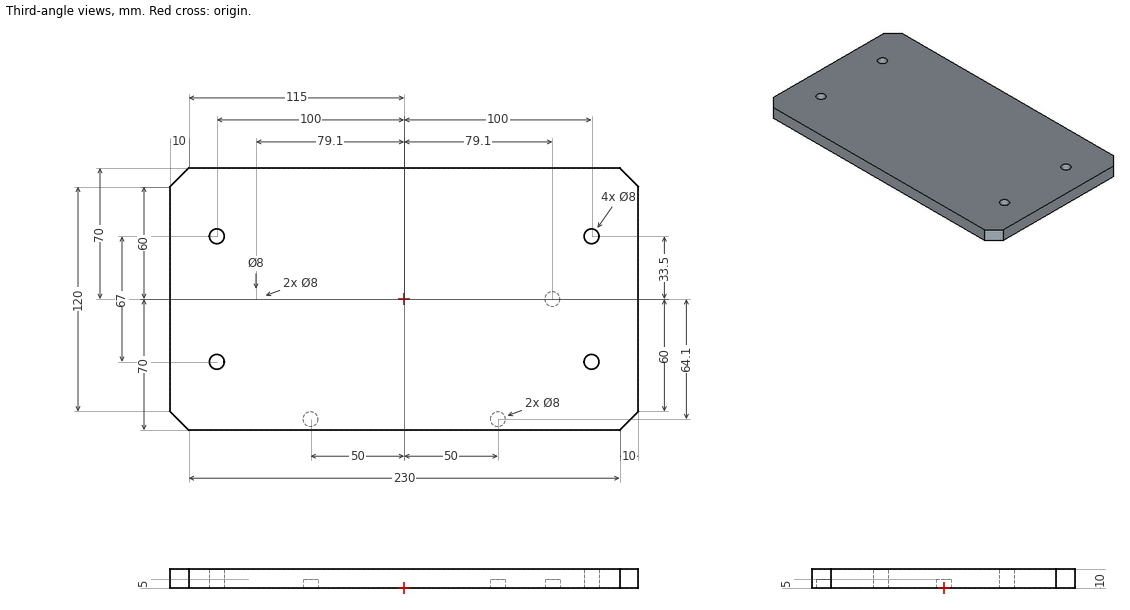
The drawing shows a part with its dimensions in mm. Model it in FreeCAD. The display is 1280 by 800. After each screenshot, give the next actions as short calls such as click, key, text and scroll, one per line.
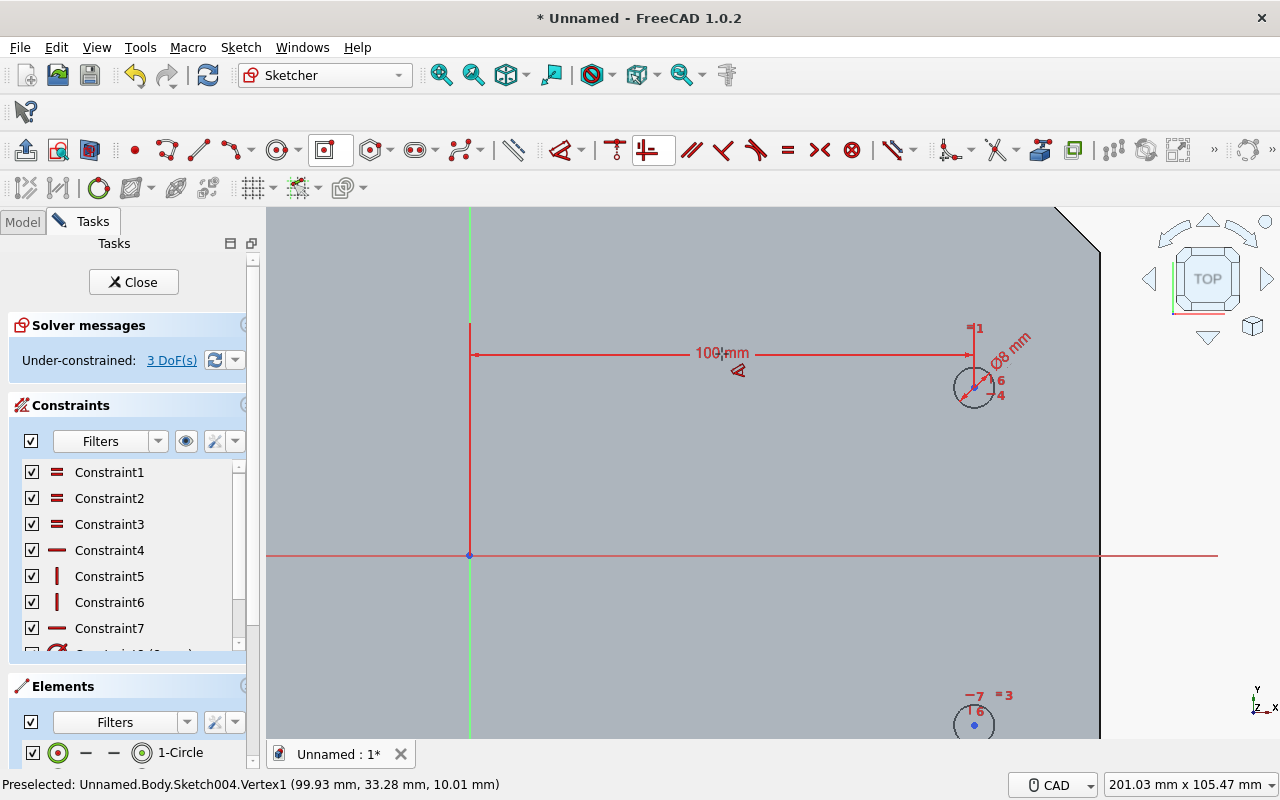
scroll(990, 373, down, 3)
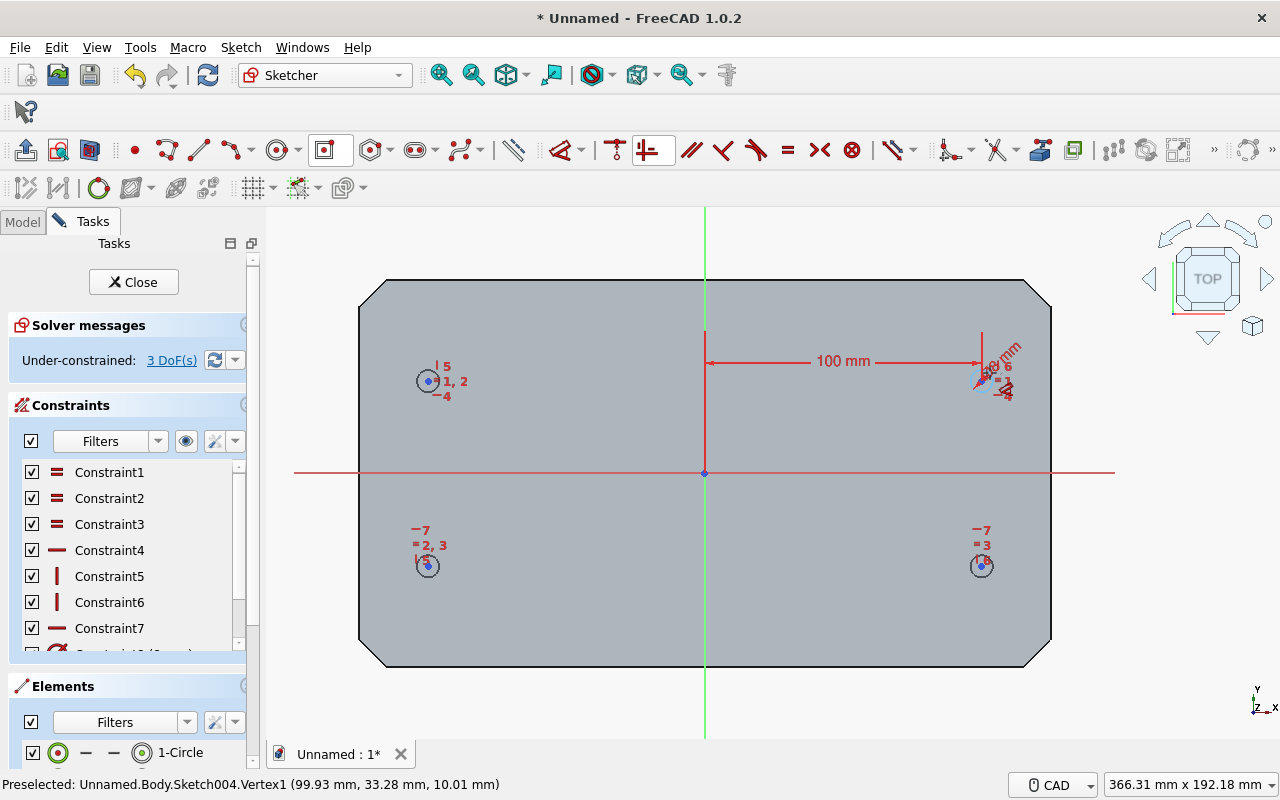
click(428, 381)
click(566, 347)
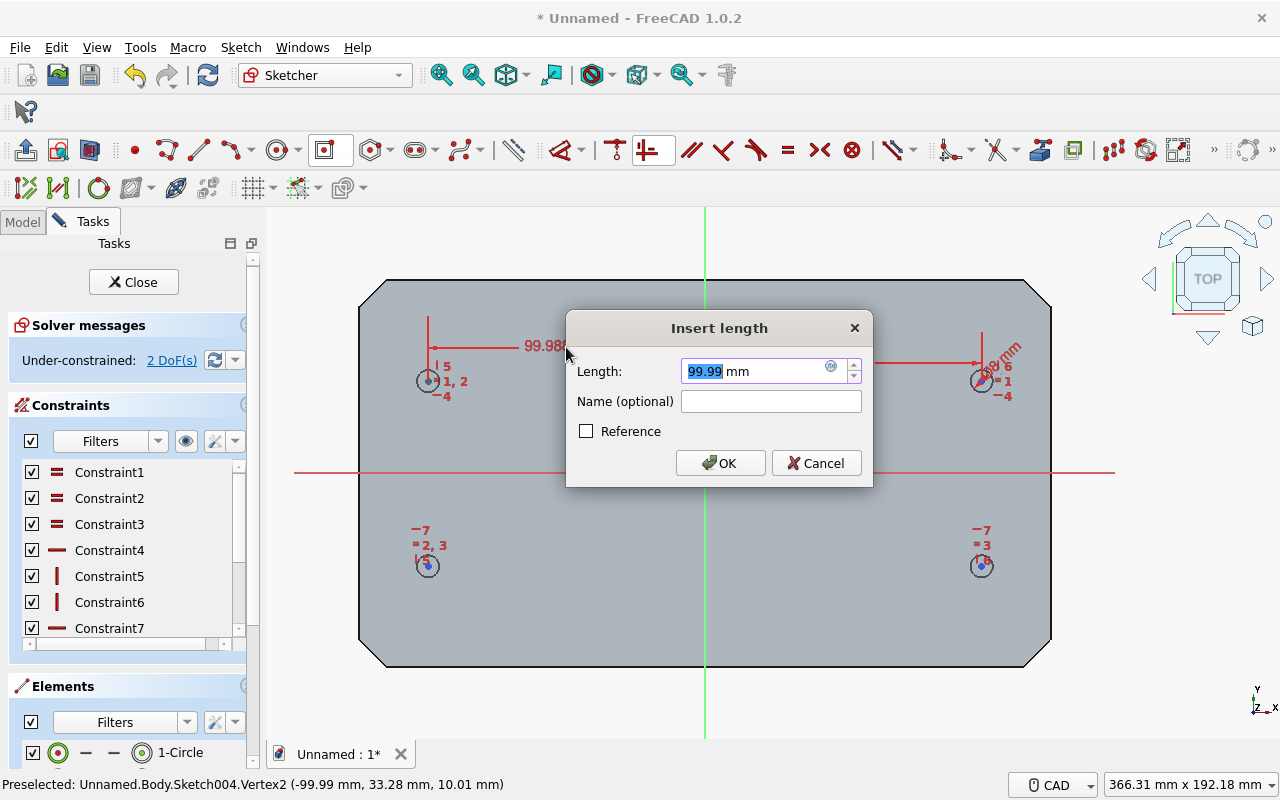
text(100)
key(Return)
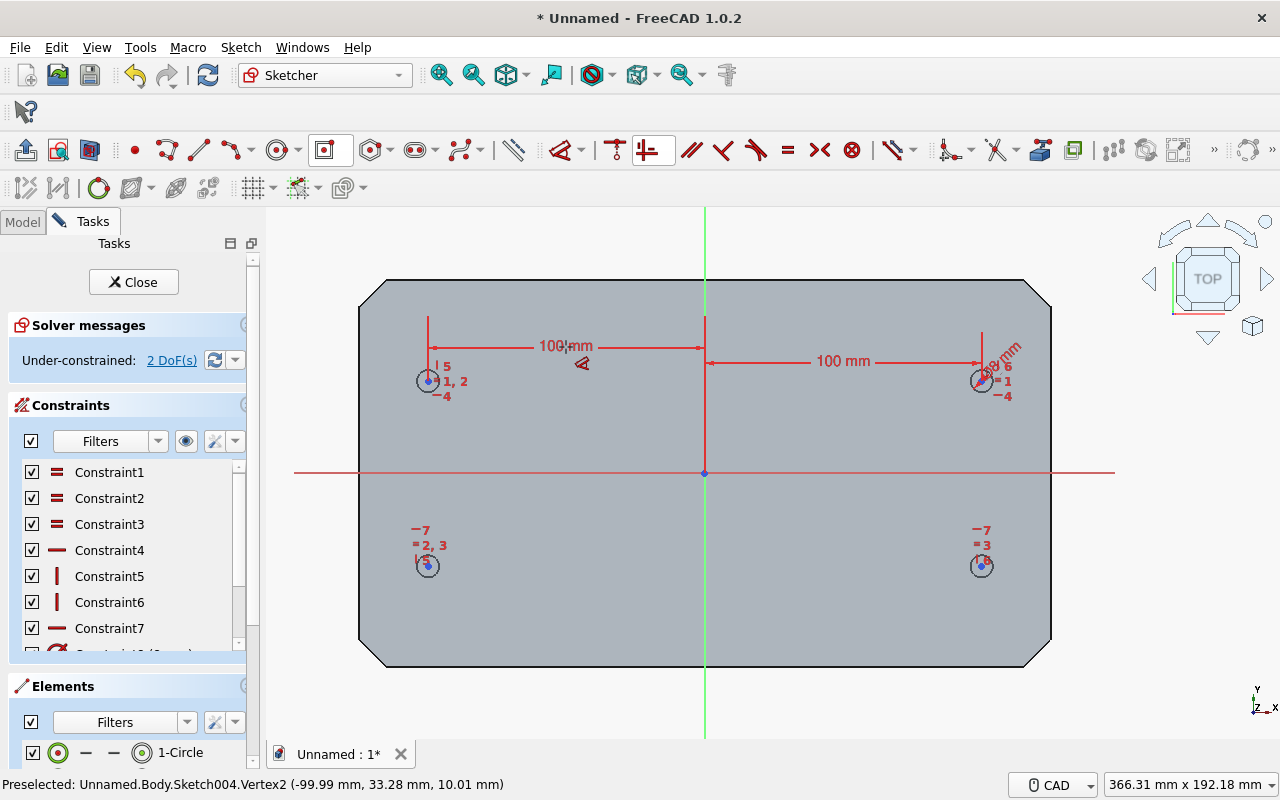
click(428, 381)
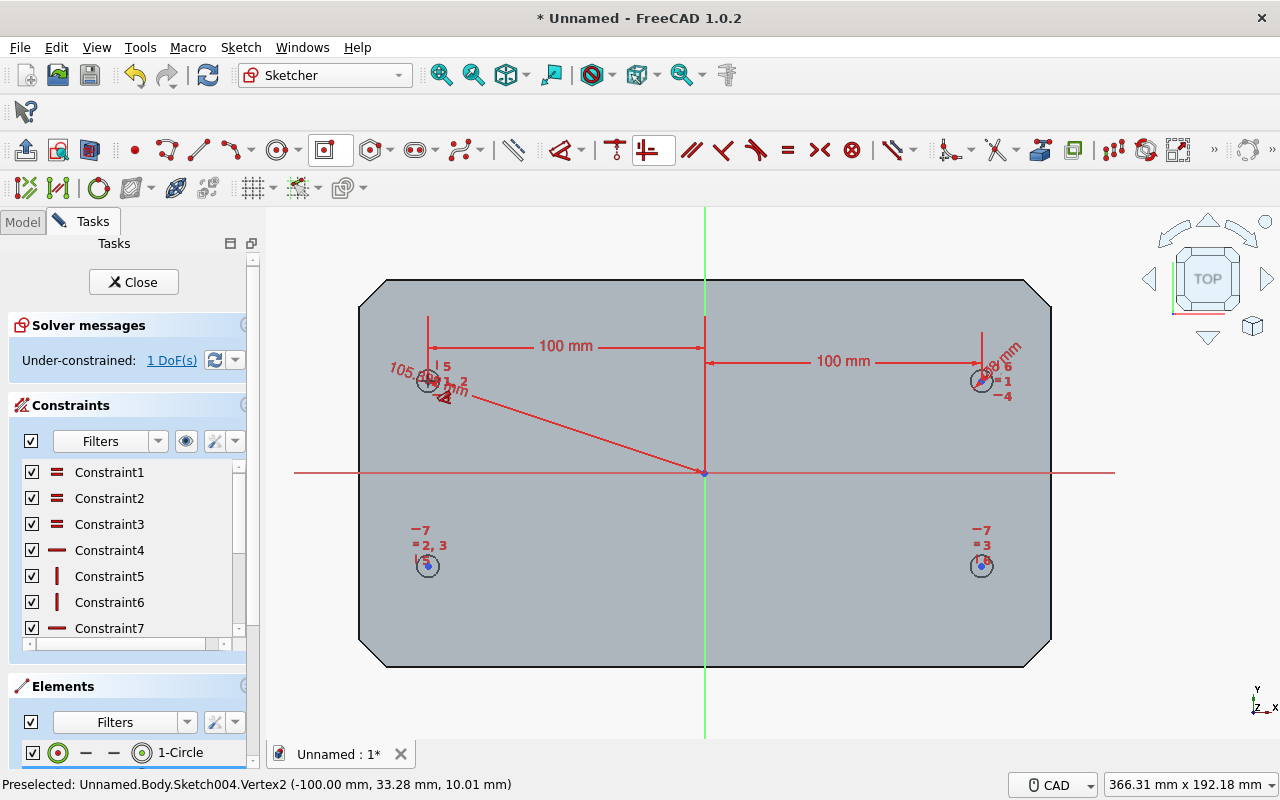
click(428, 566)
click(394, 431)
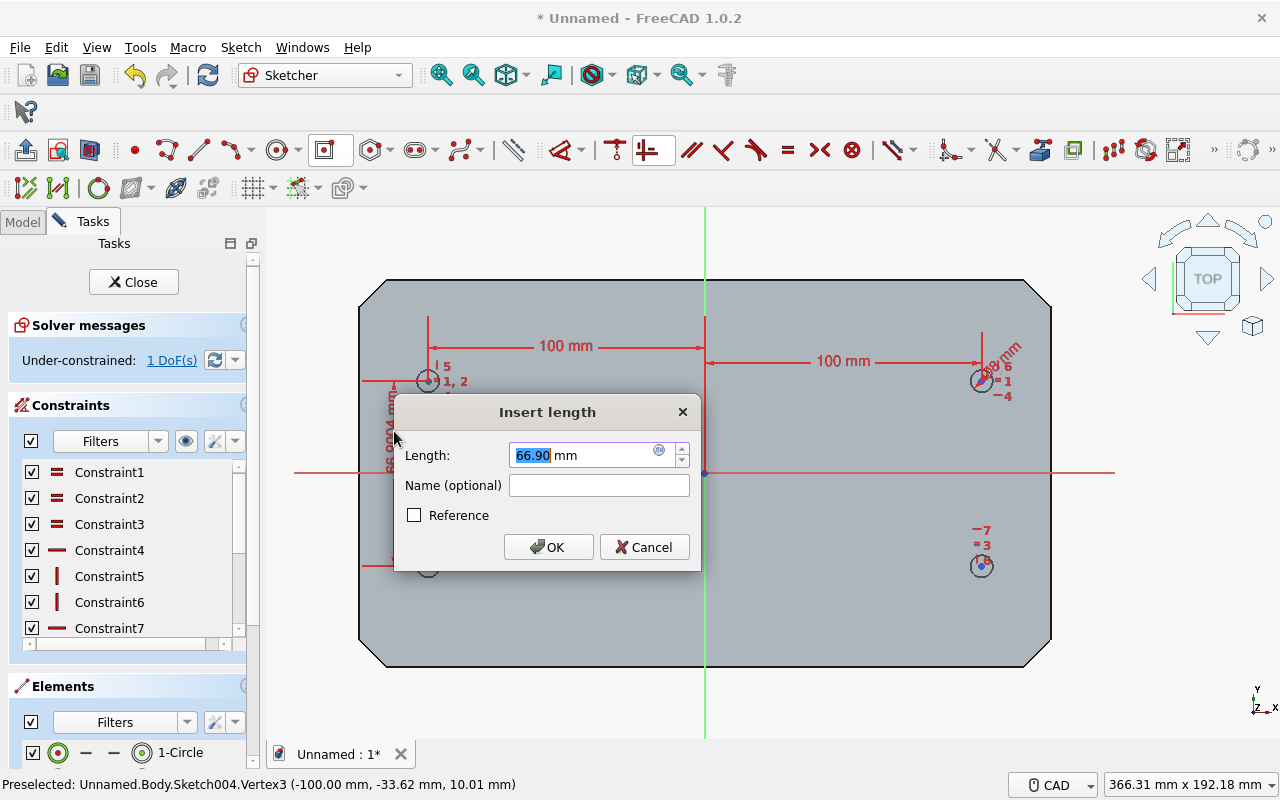
text(67)
key(Return)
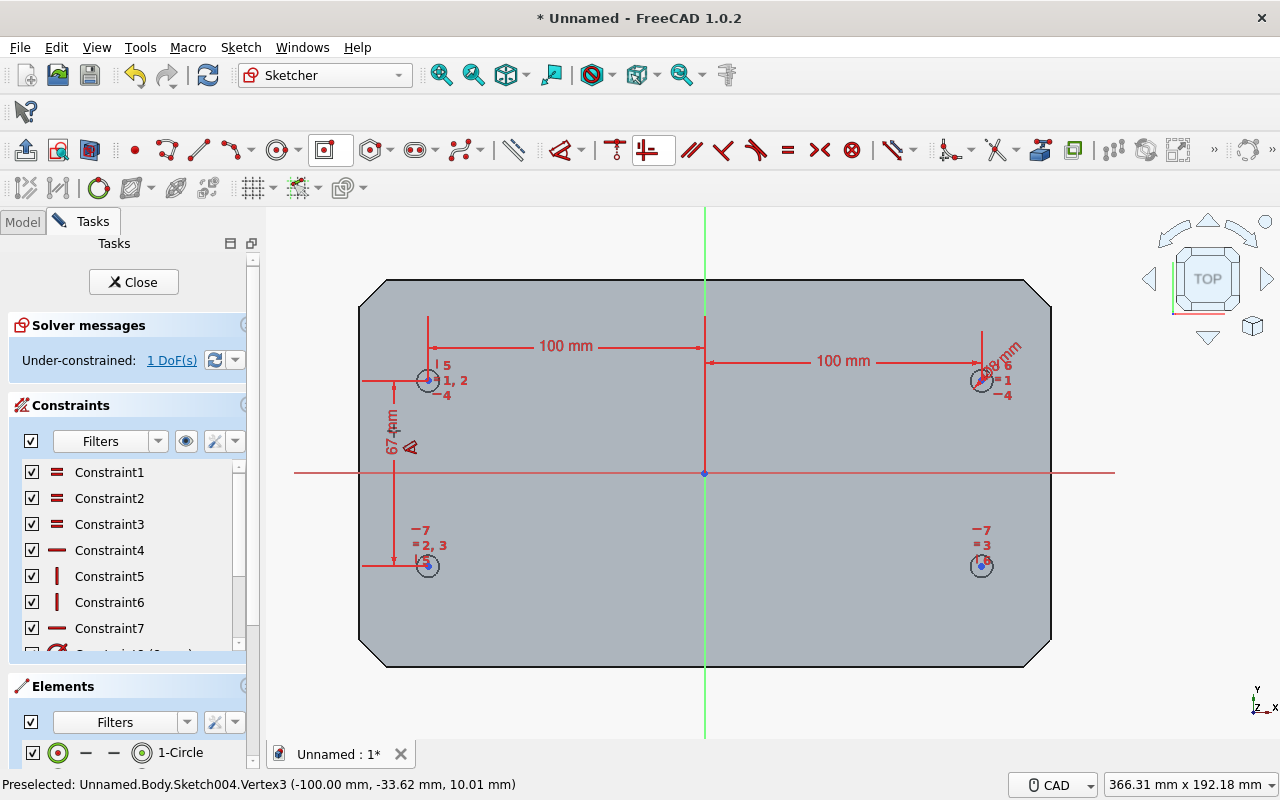
click(982, 381)
click(1016, 427)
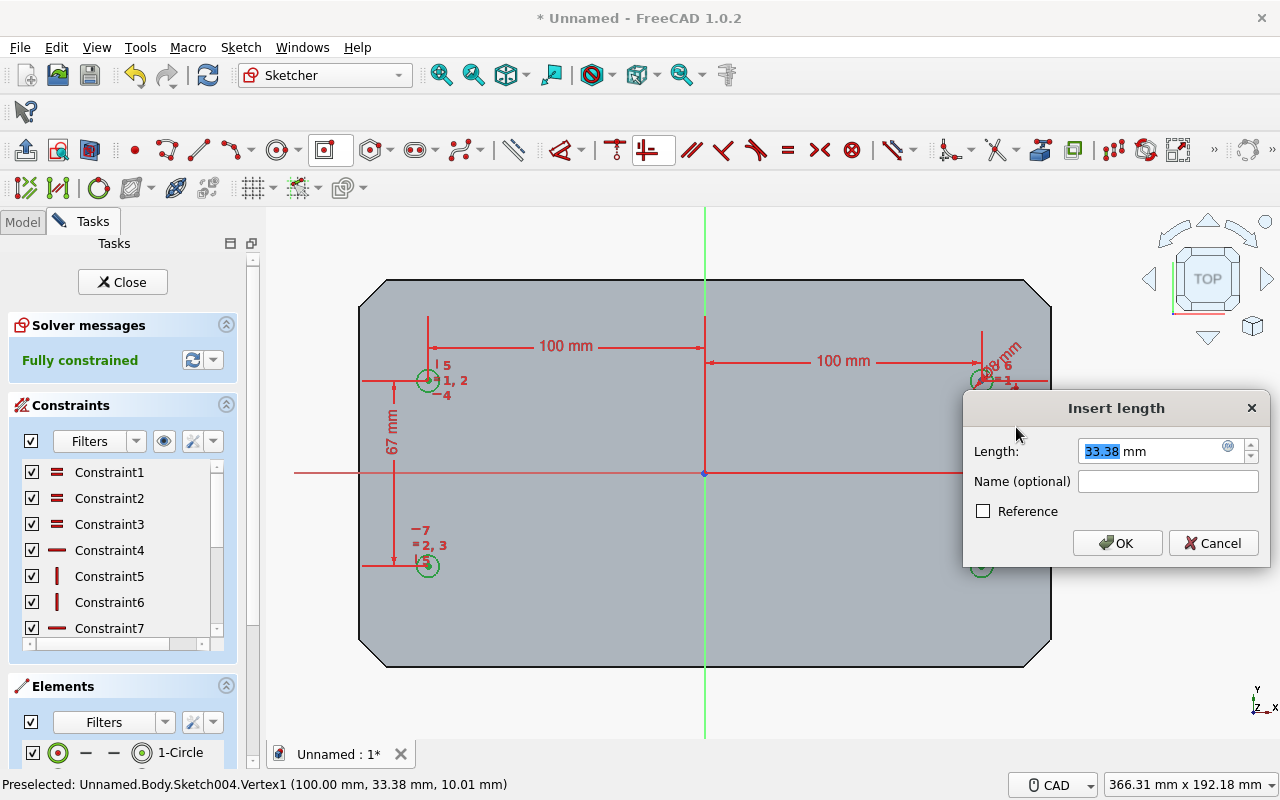
text(33.5)
key(Return)
key(Escape)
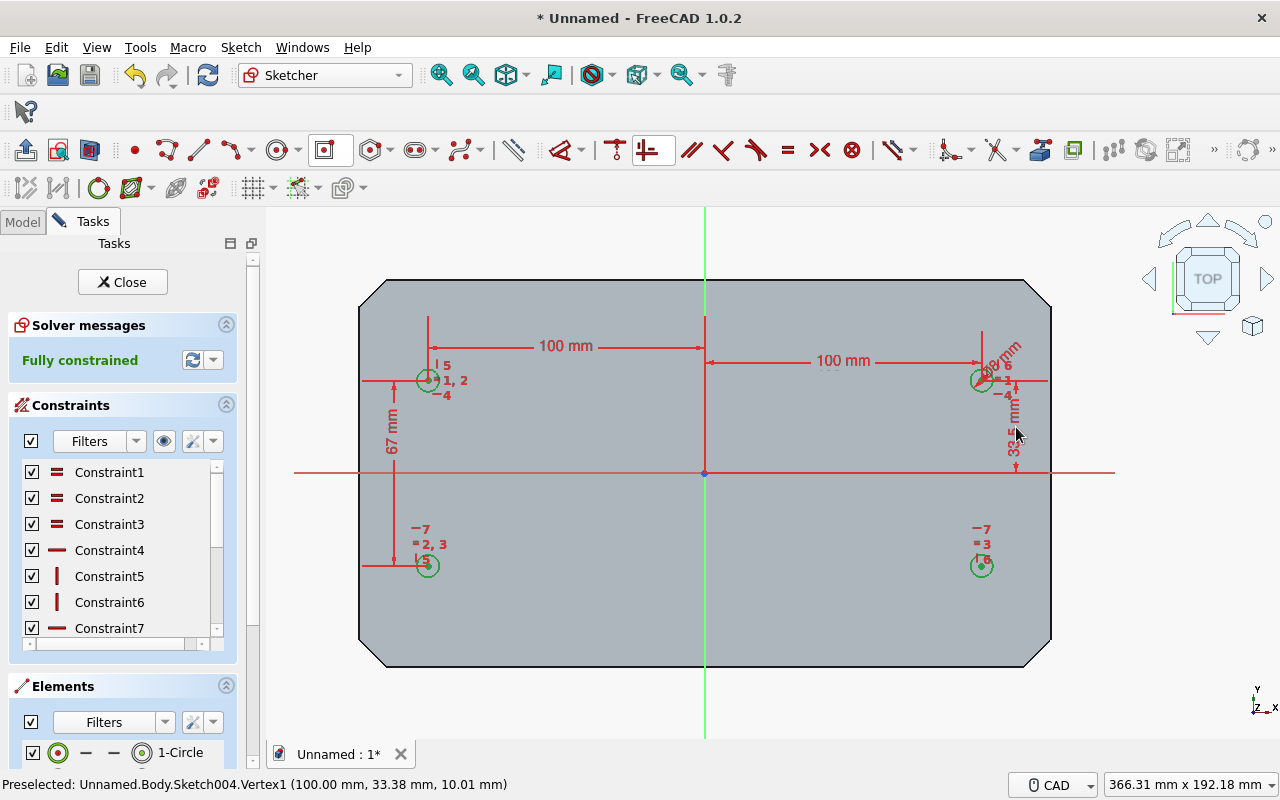
click(123, 282)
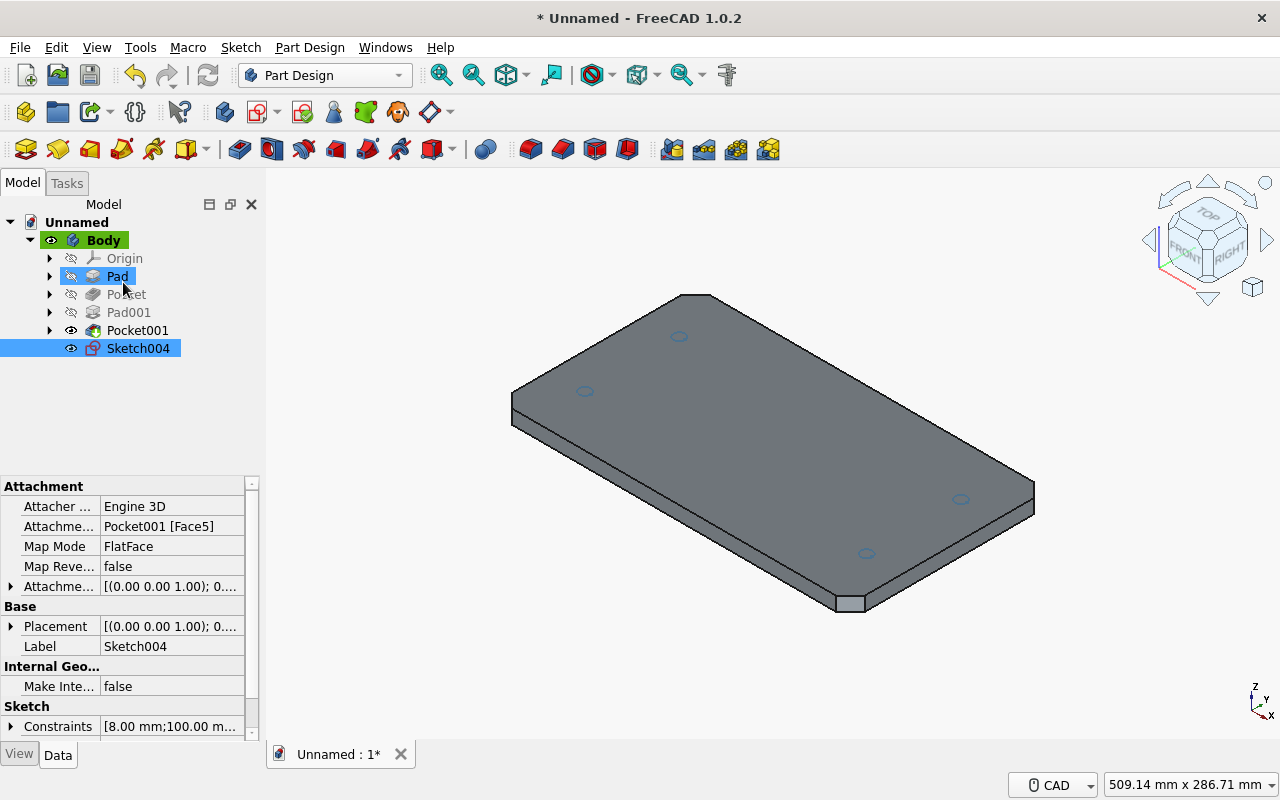
click(240, 150)